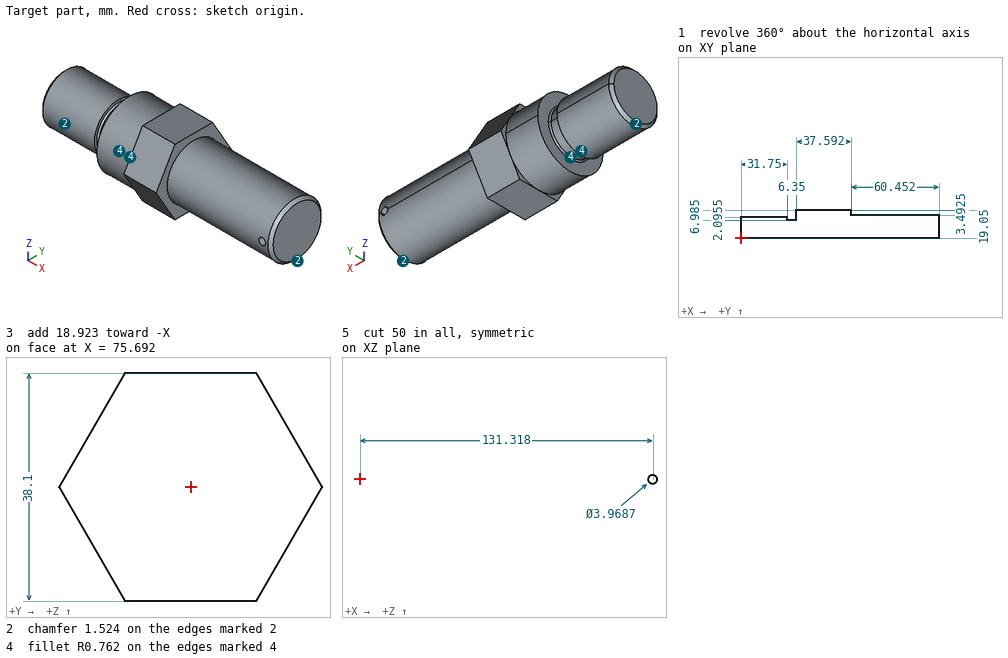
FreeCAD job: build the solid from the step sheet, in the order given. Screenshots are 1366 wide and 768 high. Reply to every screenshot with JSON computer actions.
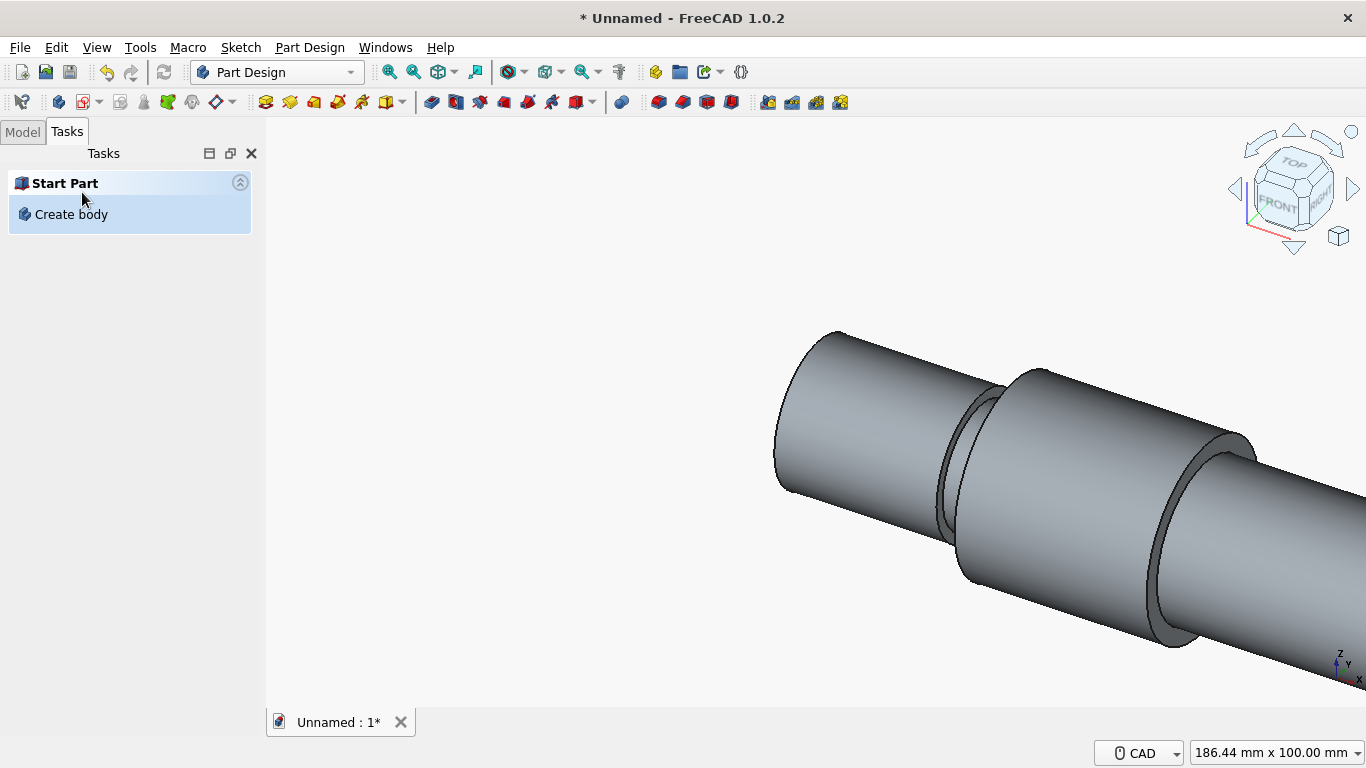
{"action": "key", "text": "v f"}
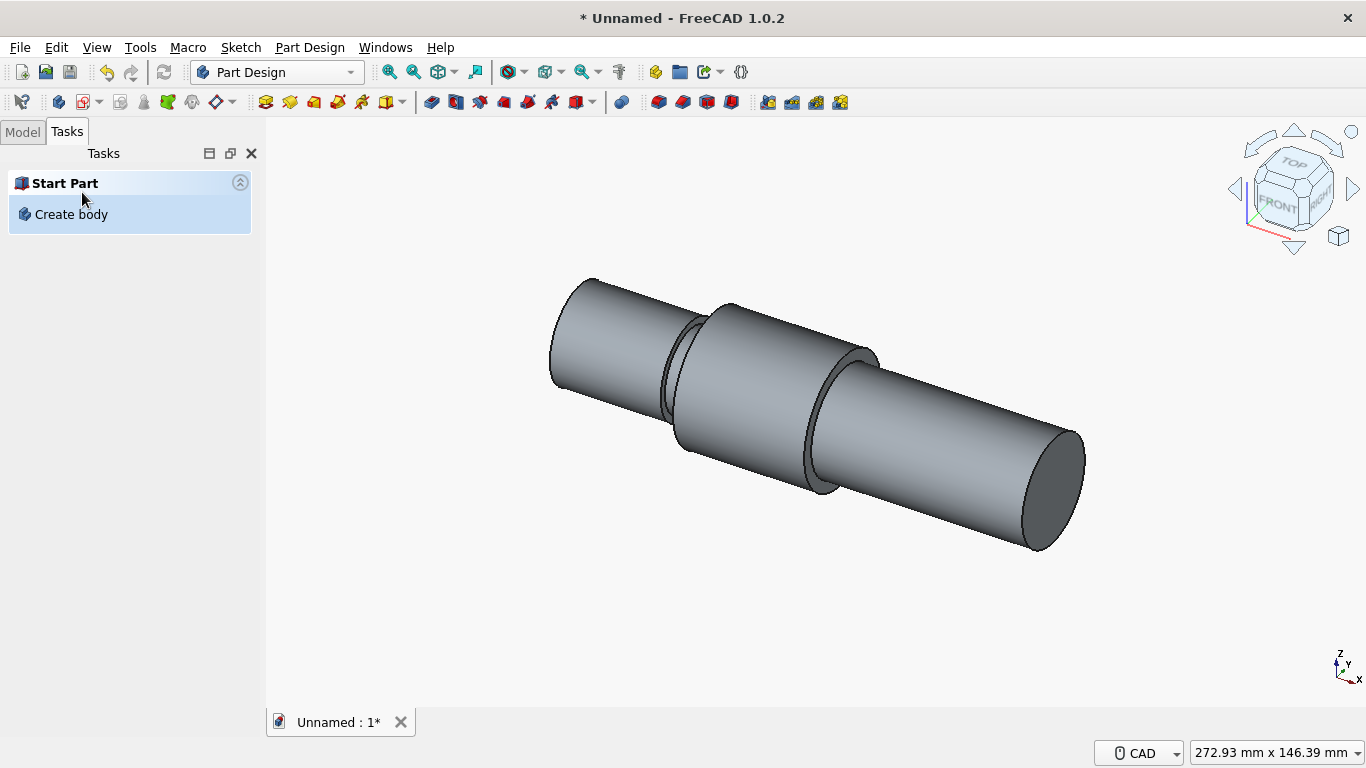
{"action": "left_click", "coordinate": [1022, 521]}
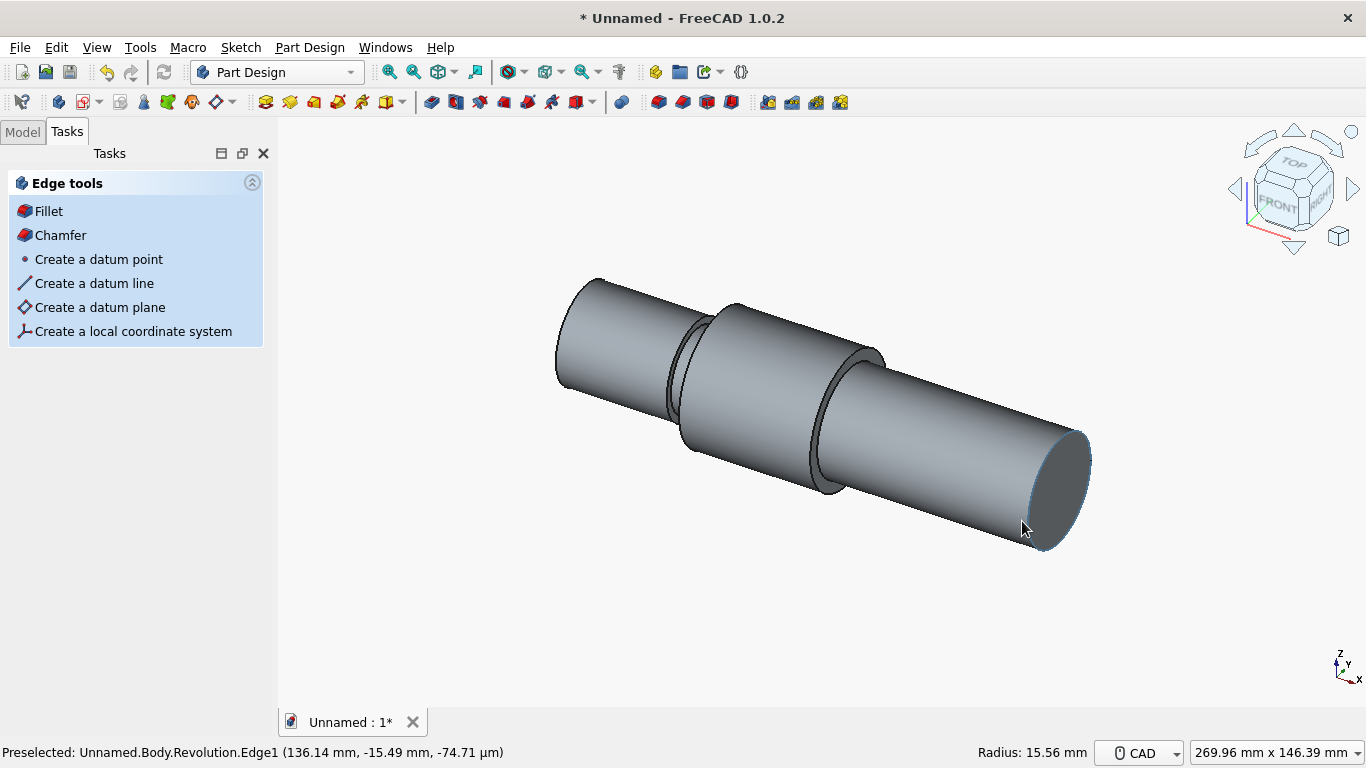
{"action": "key", "text": "0"}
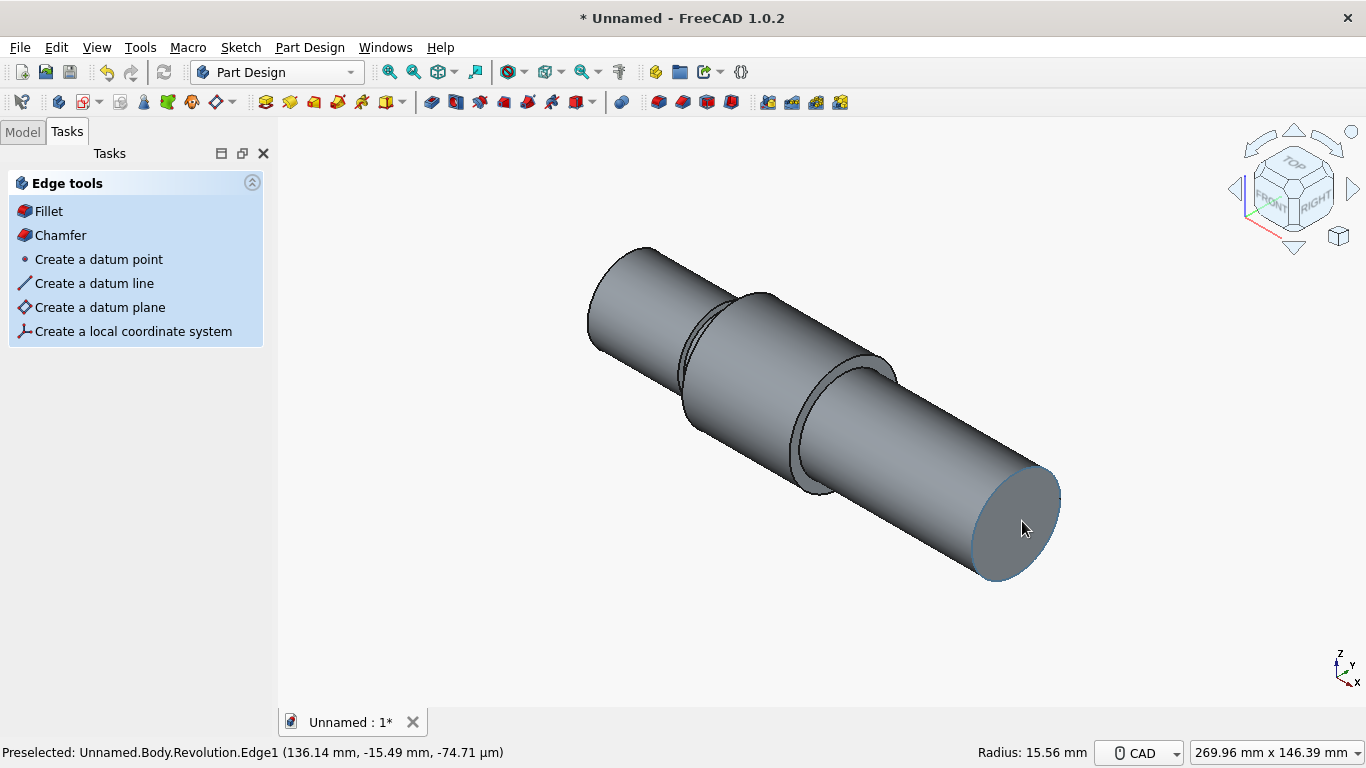
{"action": "left_click", "coordinate": [615, 262], "text": "ctrl"}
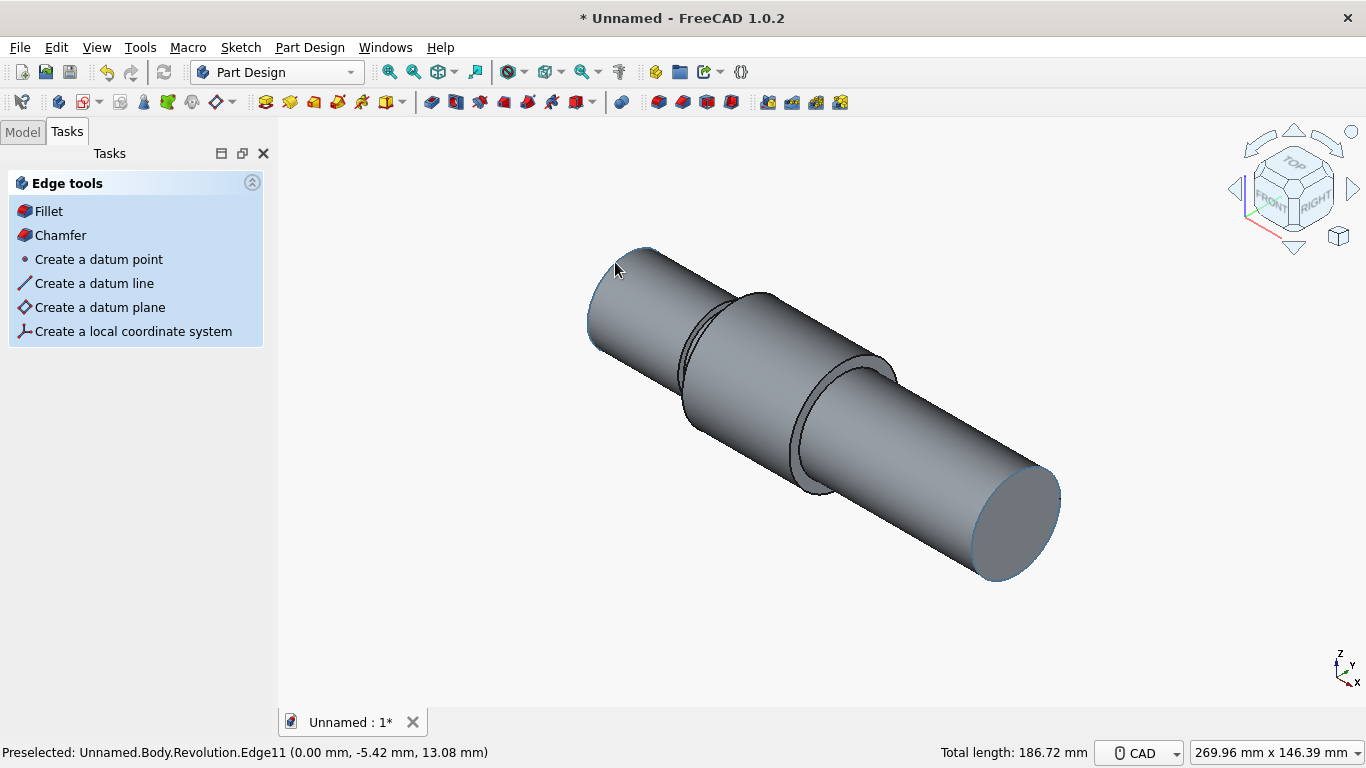
{"action": "left_click", "coordinate": [684, 102]}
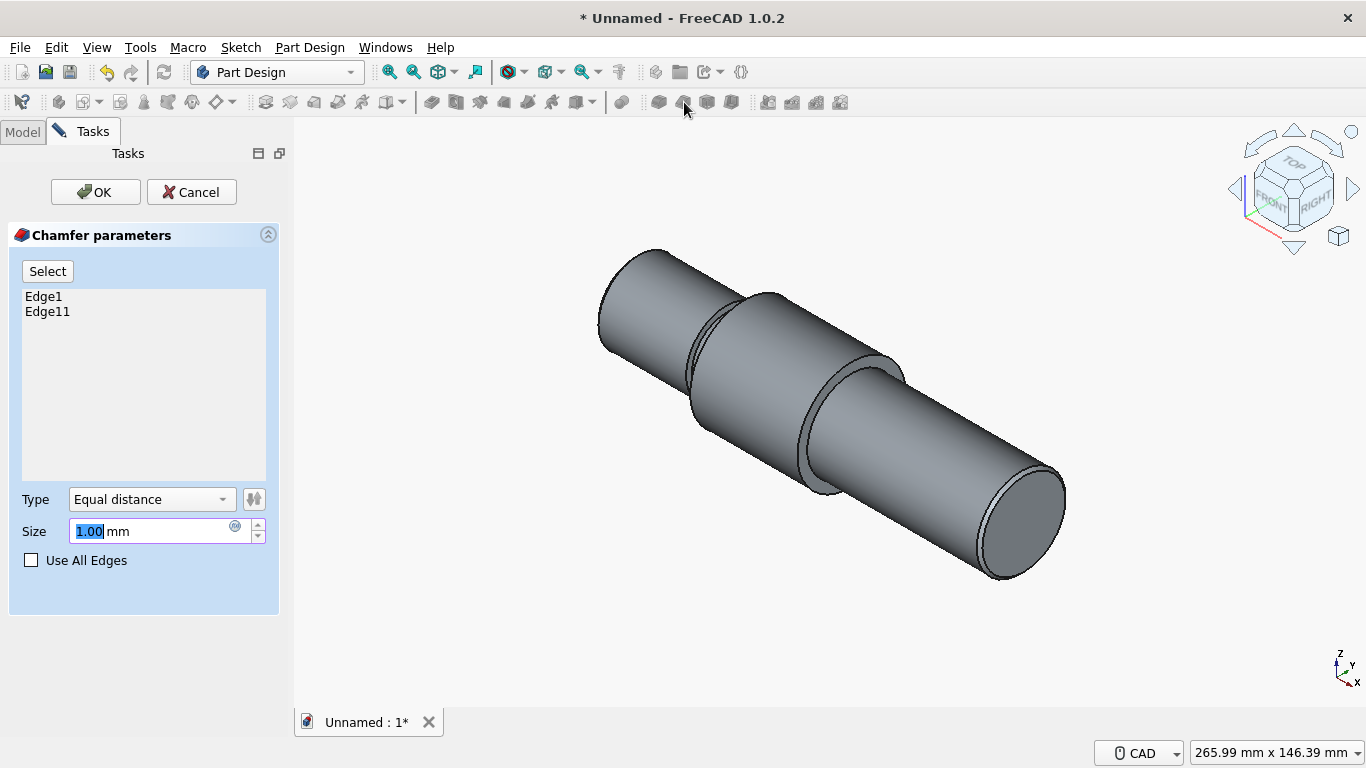
{"action": "type", "text": "1.524"}
{"action": "key", "text": "Tab"}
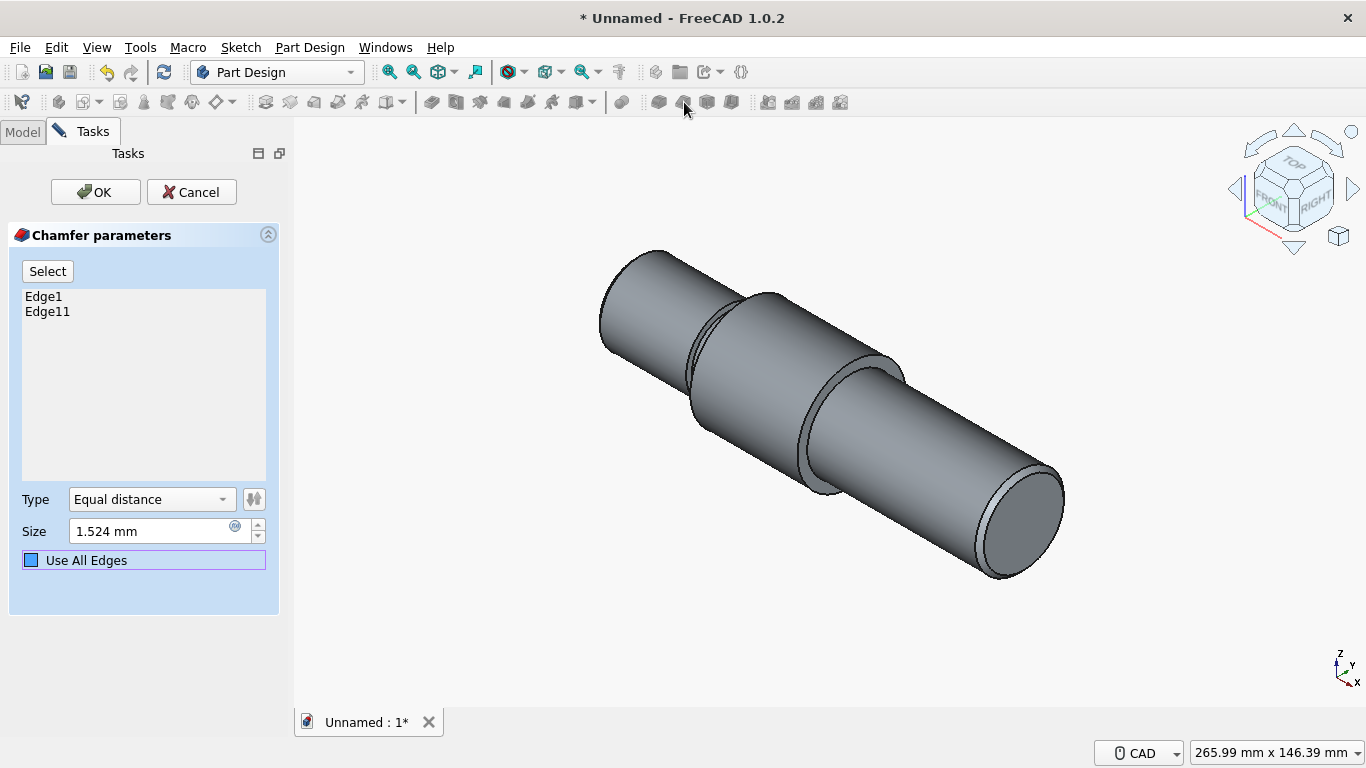
{"action": "left_click", "coordinate": [96, 192]}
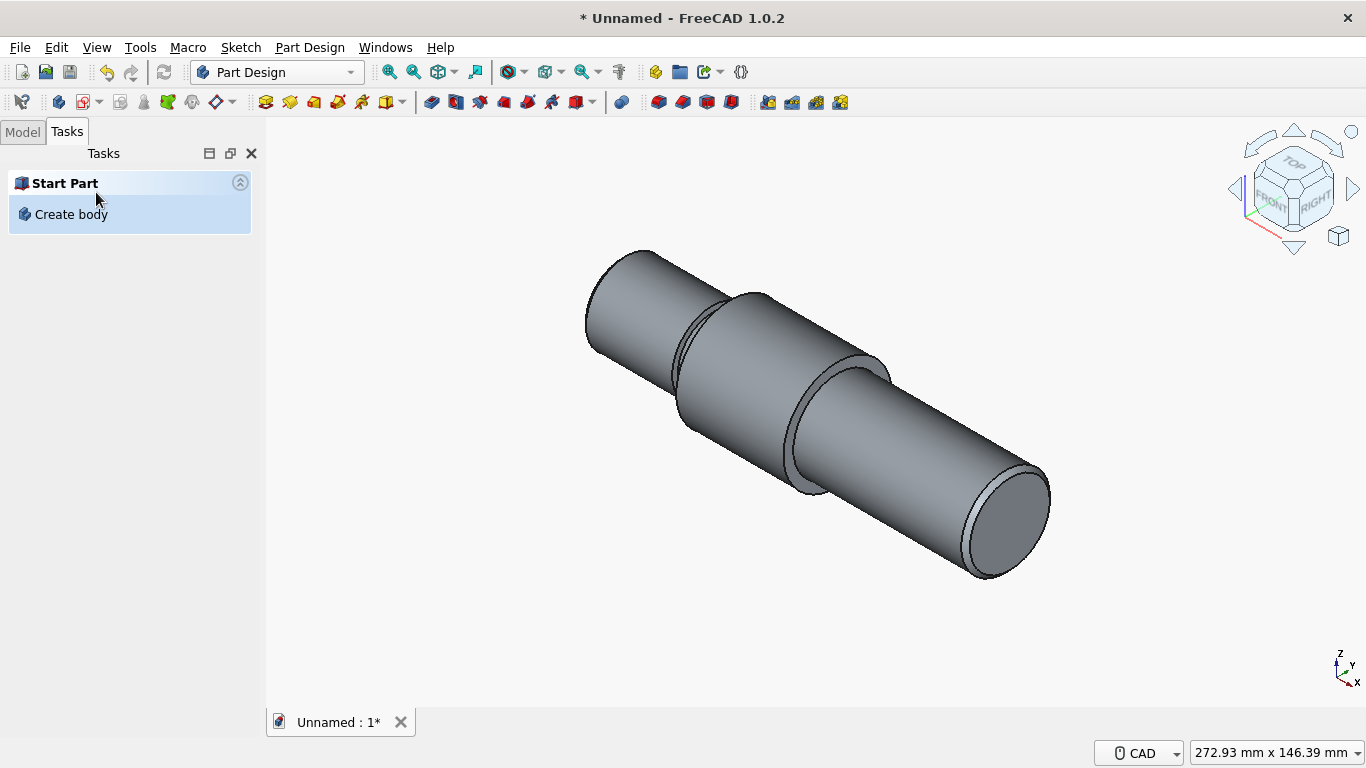
{"action": "scroll", "coordinate": [884, 379], "scroll_direction": "up", "scroll_amount": 3}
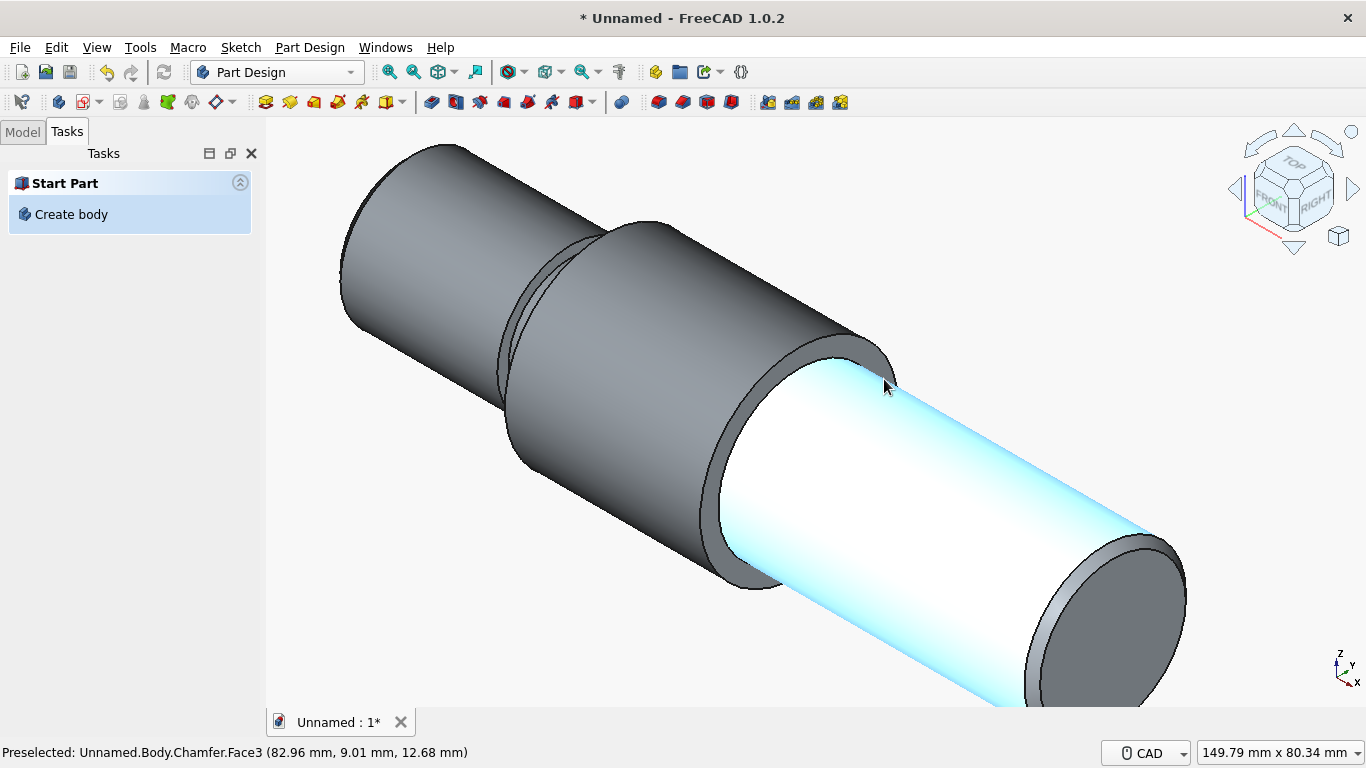
{"action": "left_click", "coordinate": [827, 346]}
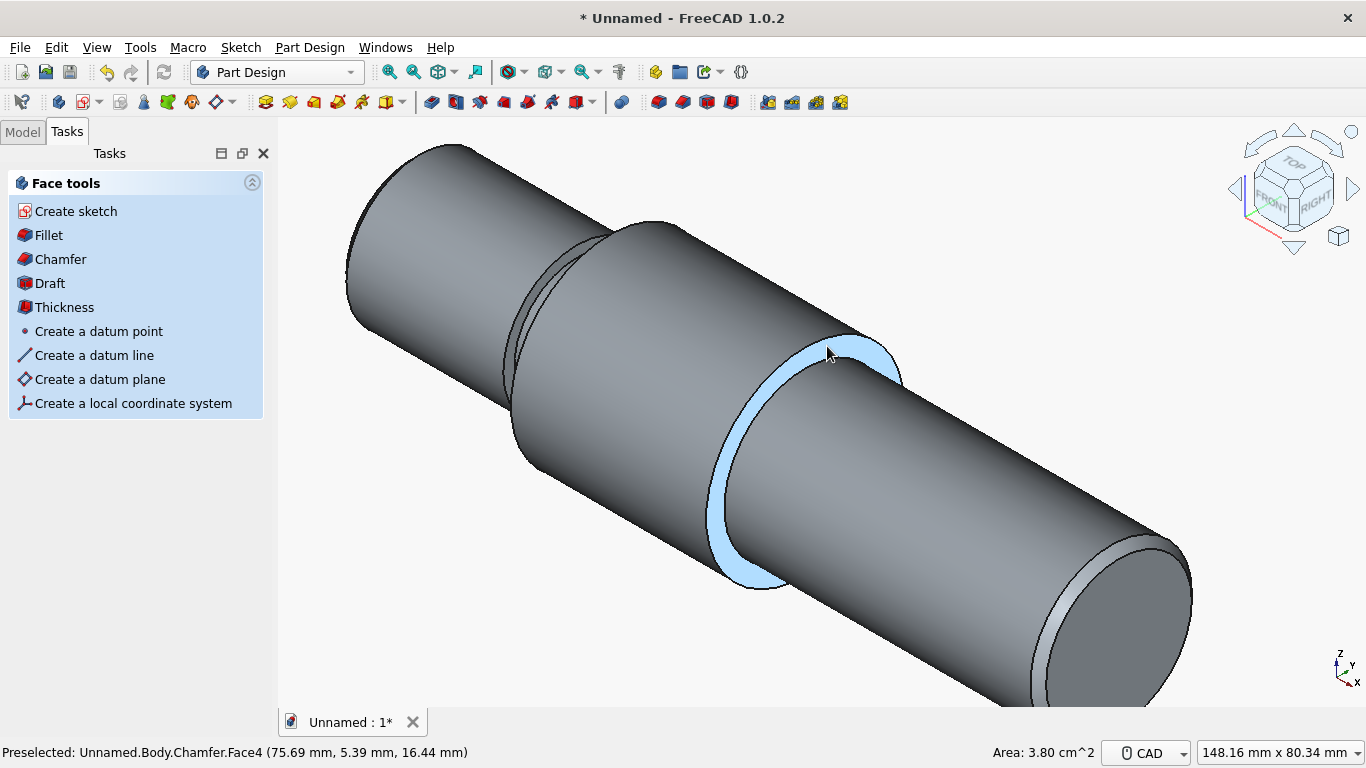
{"action": "left_click", "coordinate": [84, 102]}